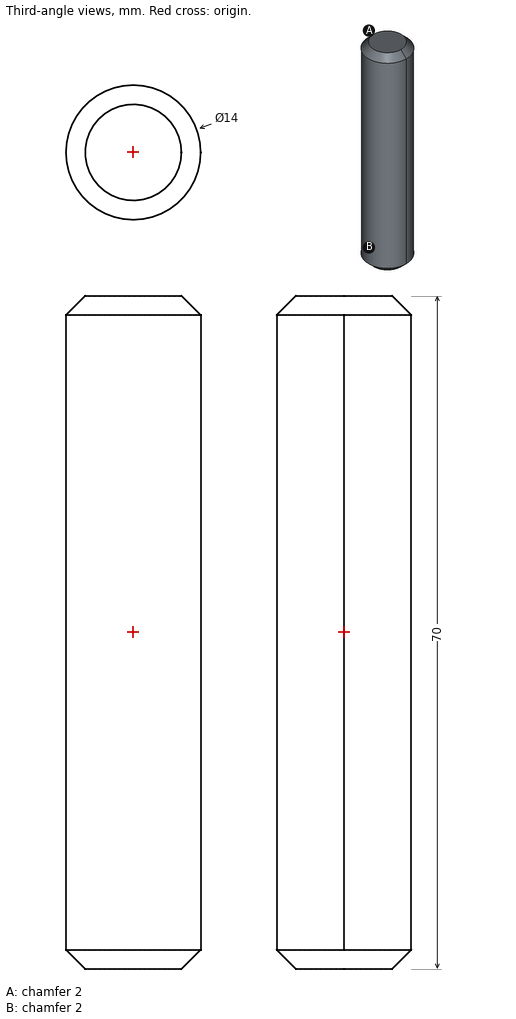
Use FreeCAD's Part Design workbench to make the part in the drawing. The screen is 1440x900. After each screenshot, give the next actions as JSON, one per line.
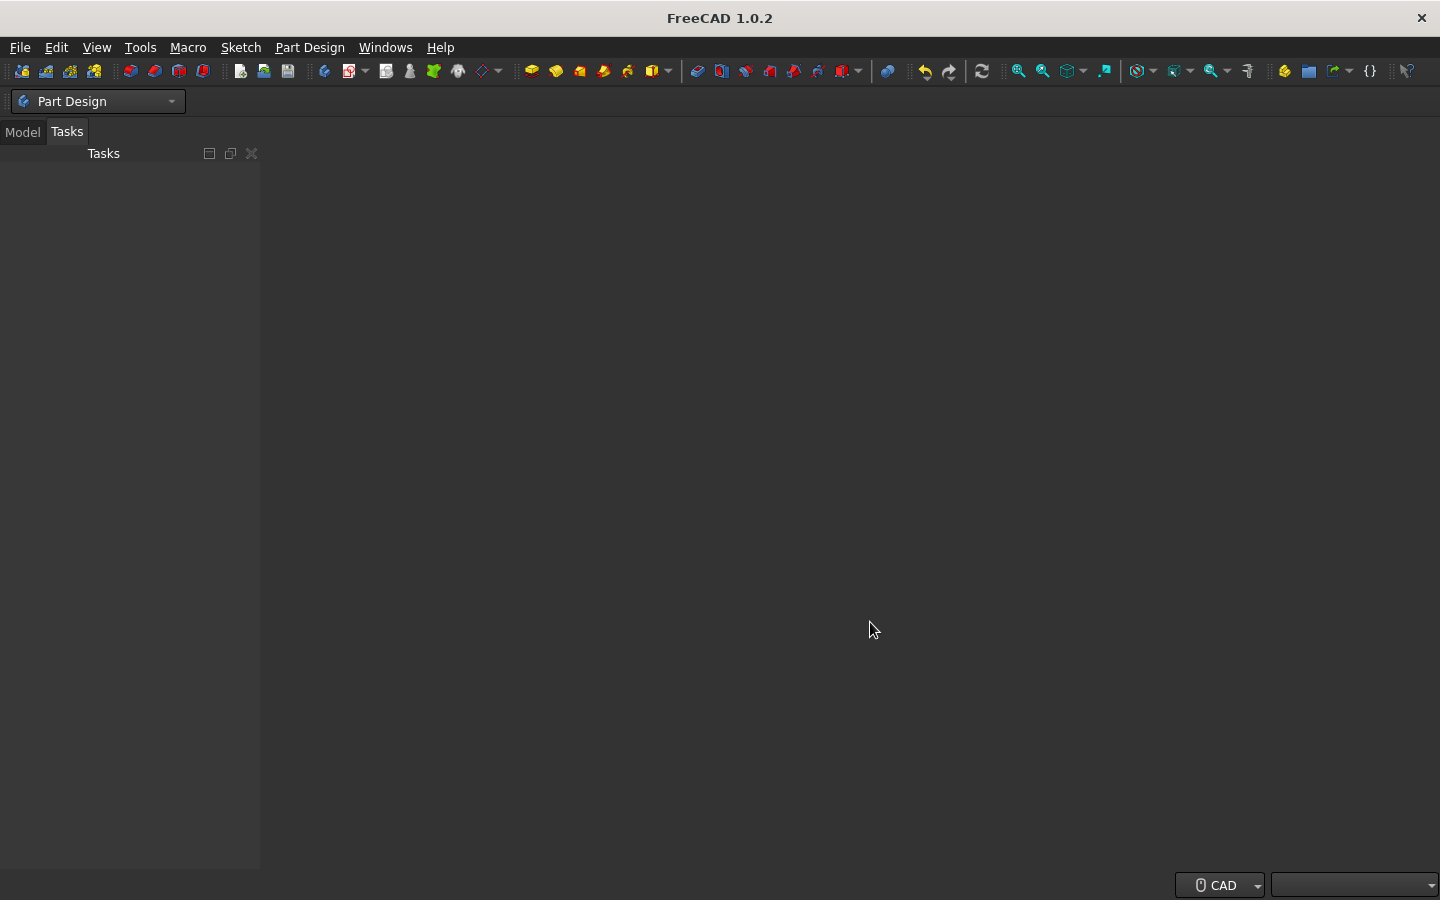
{"action": "key", "text": "ctrl+n"}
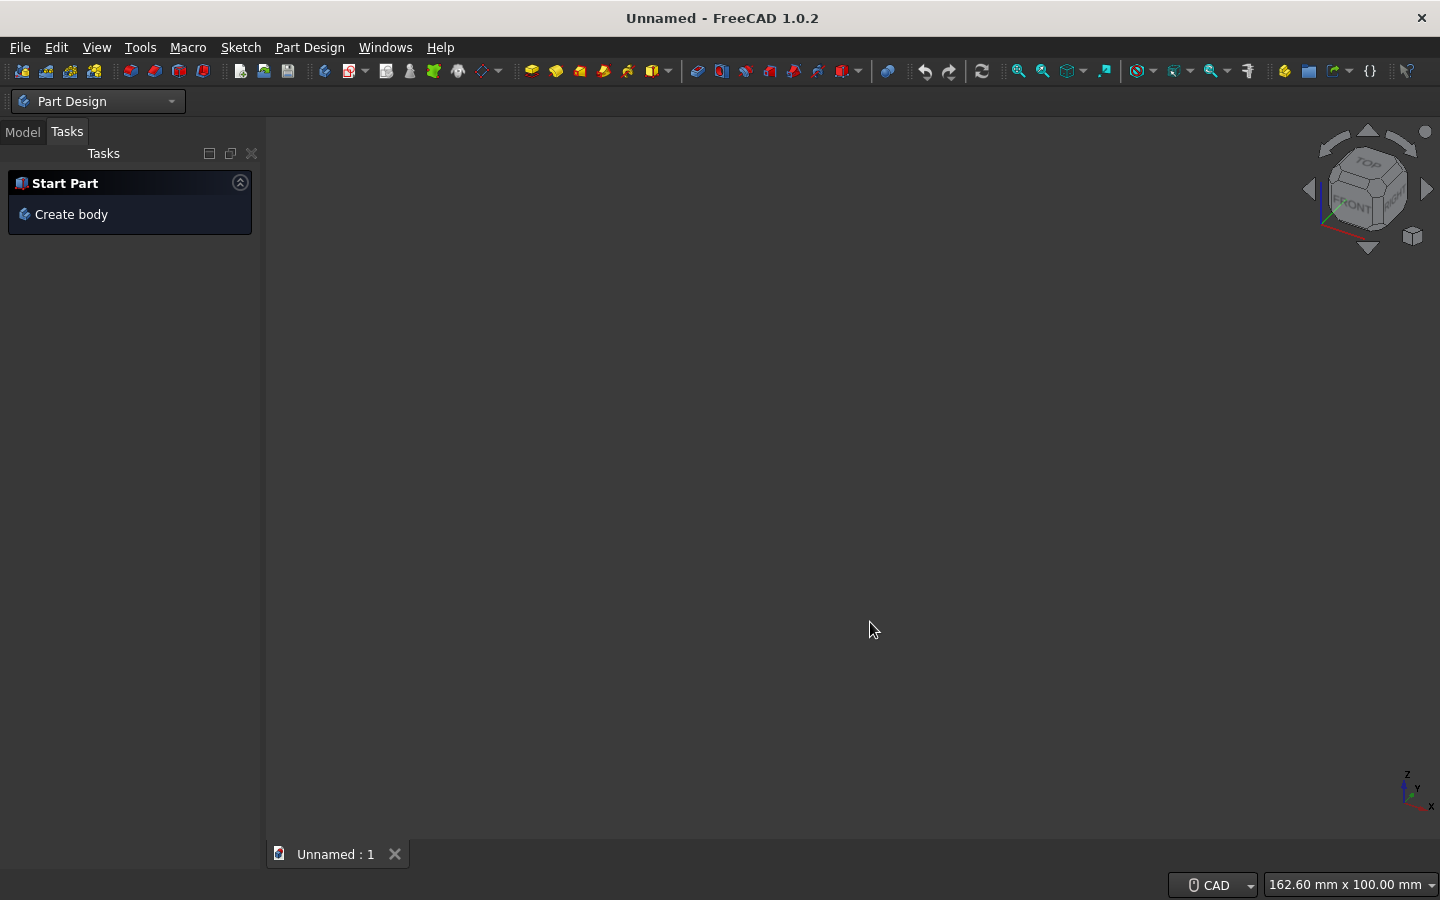
{"action": "left_click", "coordinate": [350, 72]}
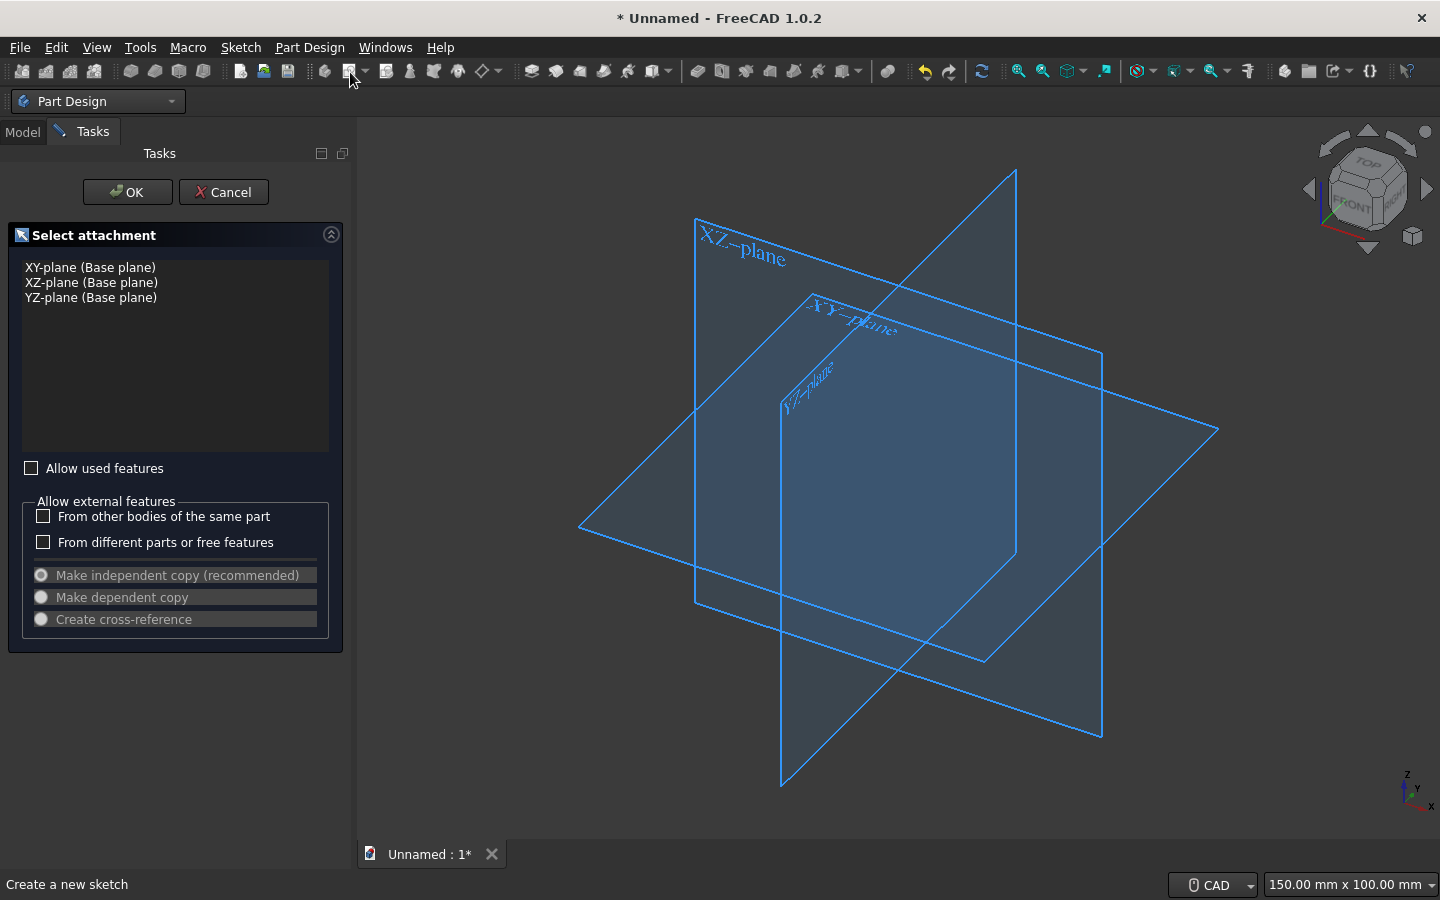
{"action": "left_click", "coordinate": [82, 268]}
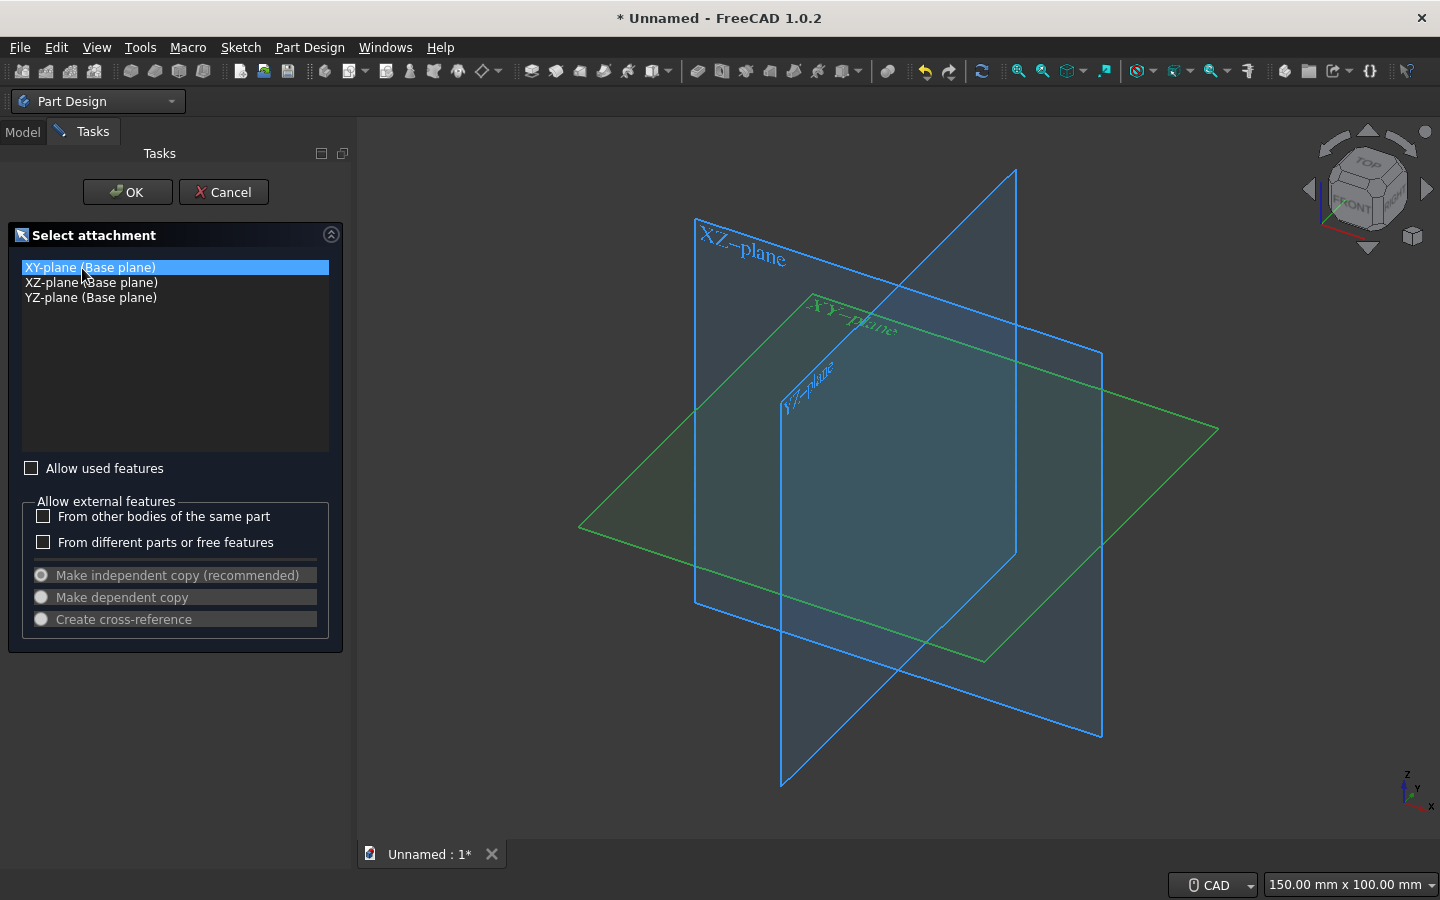
{"action": "left_click", "coordinate": [128, 192]}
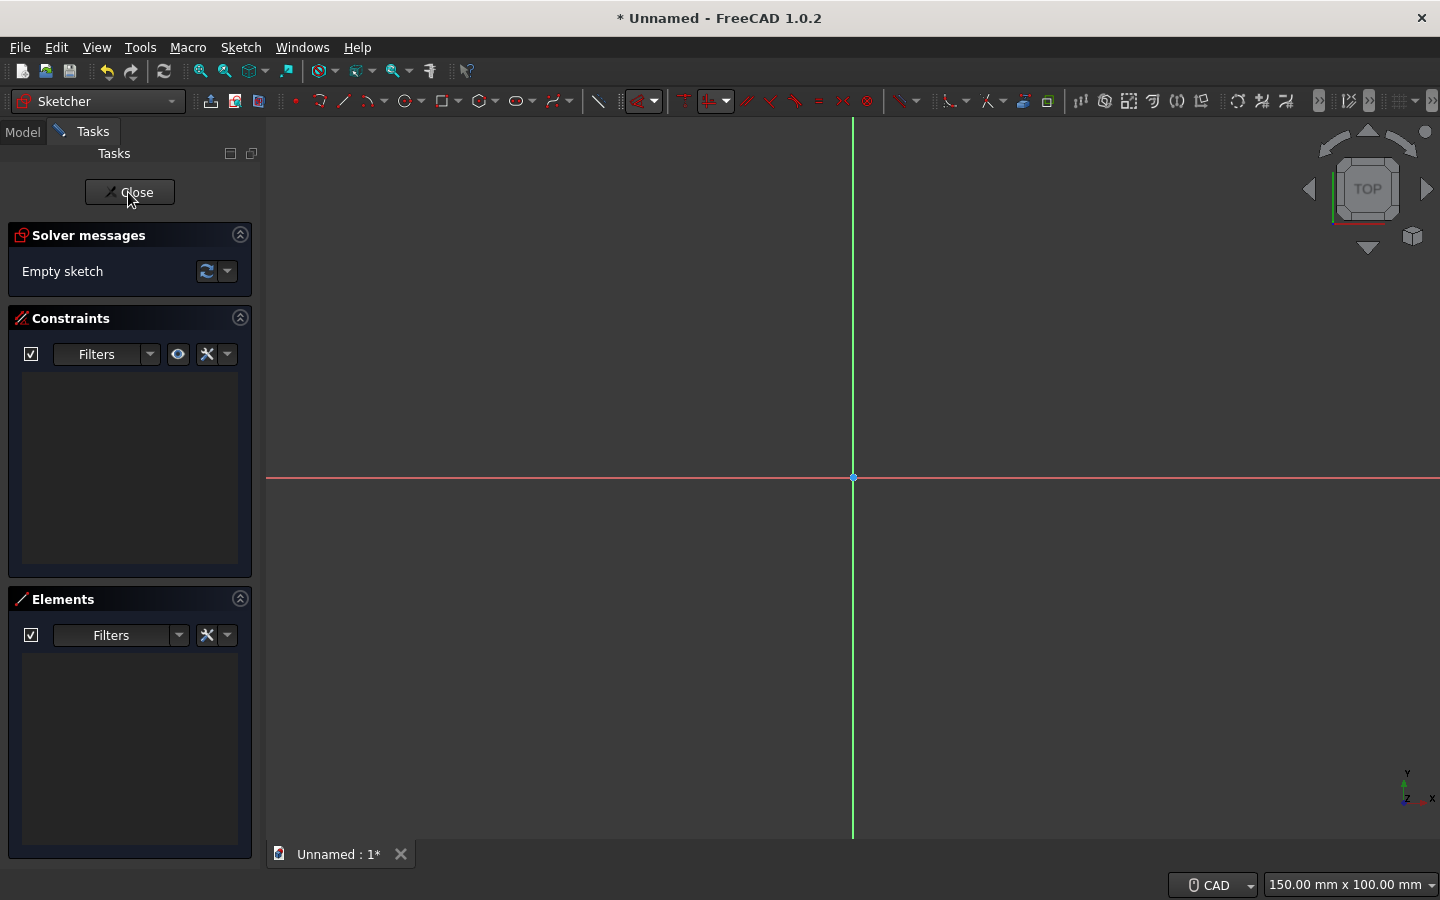
{"action": "scroll", "coordinate": [870, 478], "scroll_direction": "up", "scroll_amount": 8}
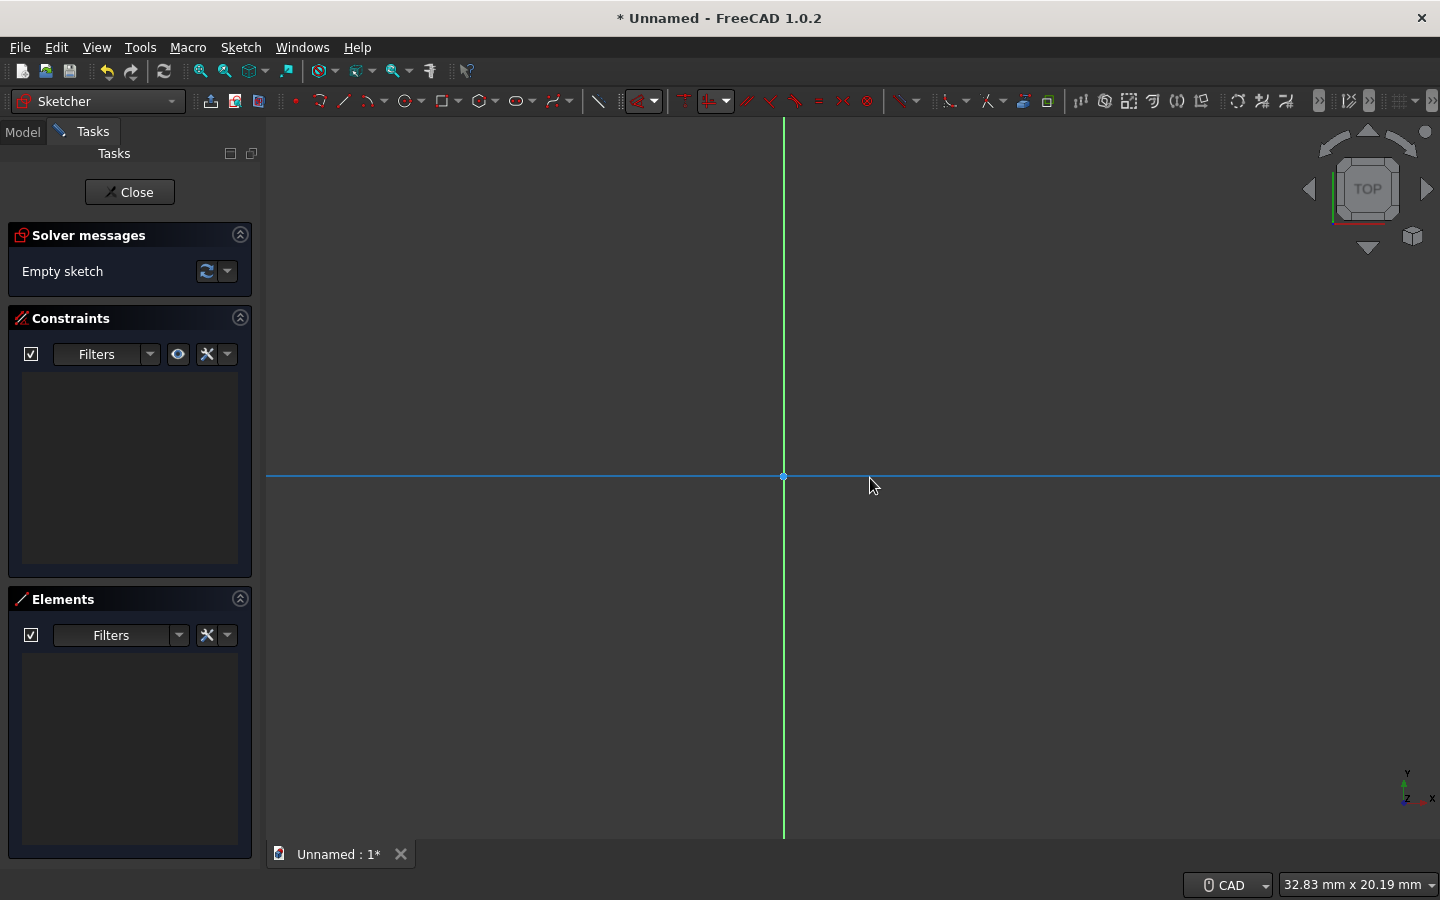
{"action": "key", "text": "g c"}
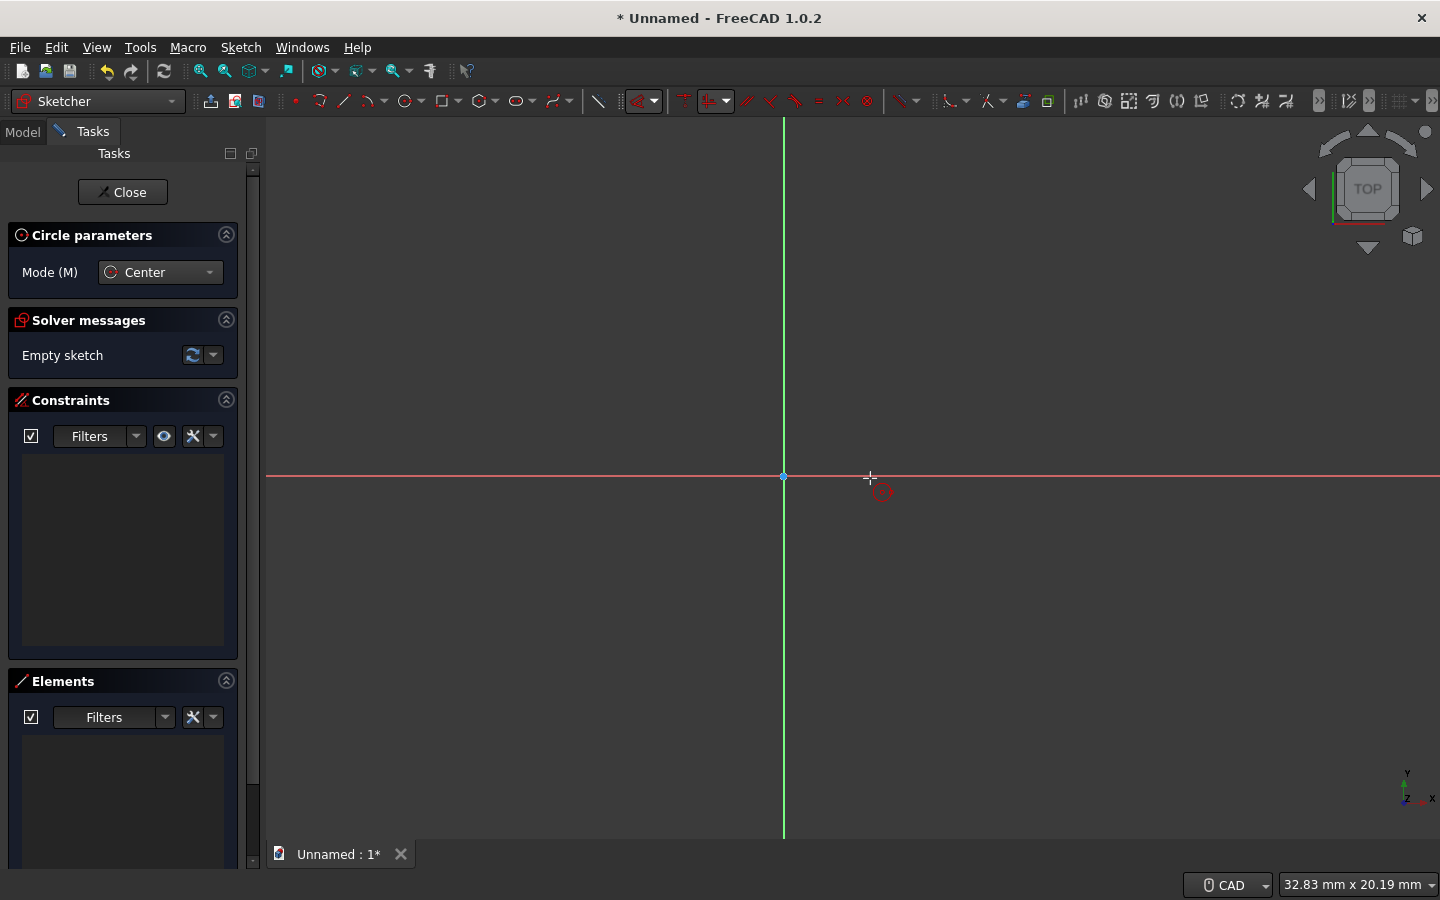
{"action": "left_click", "coordinate": [784, 476]}
{"action": "left_click", "coordinate": [961, 299]}
{"action": "key", "text": "Escape"}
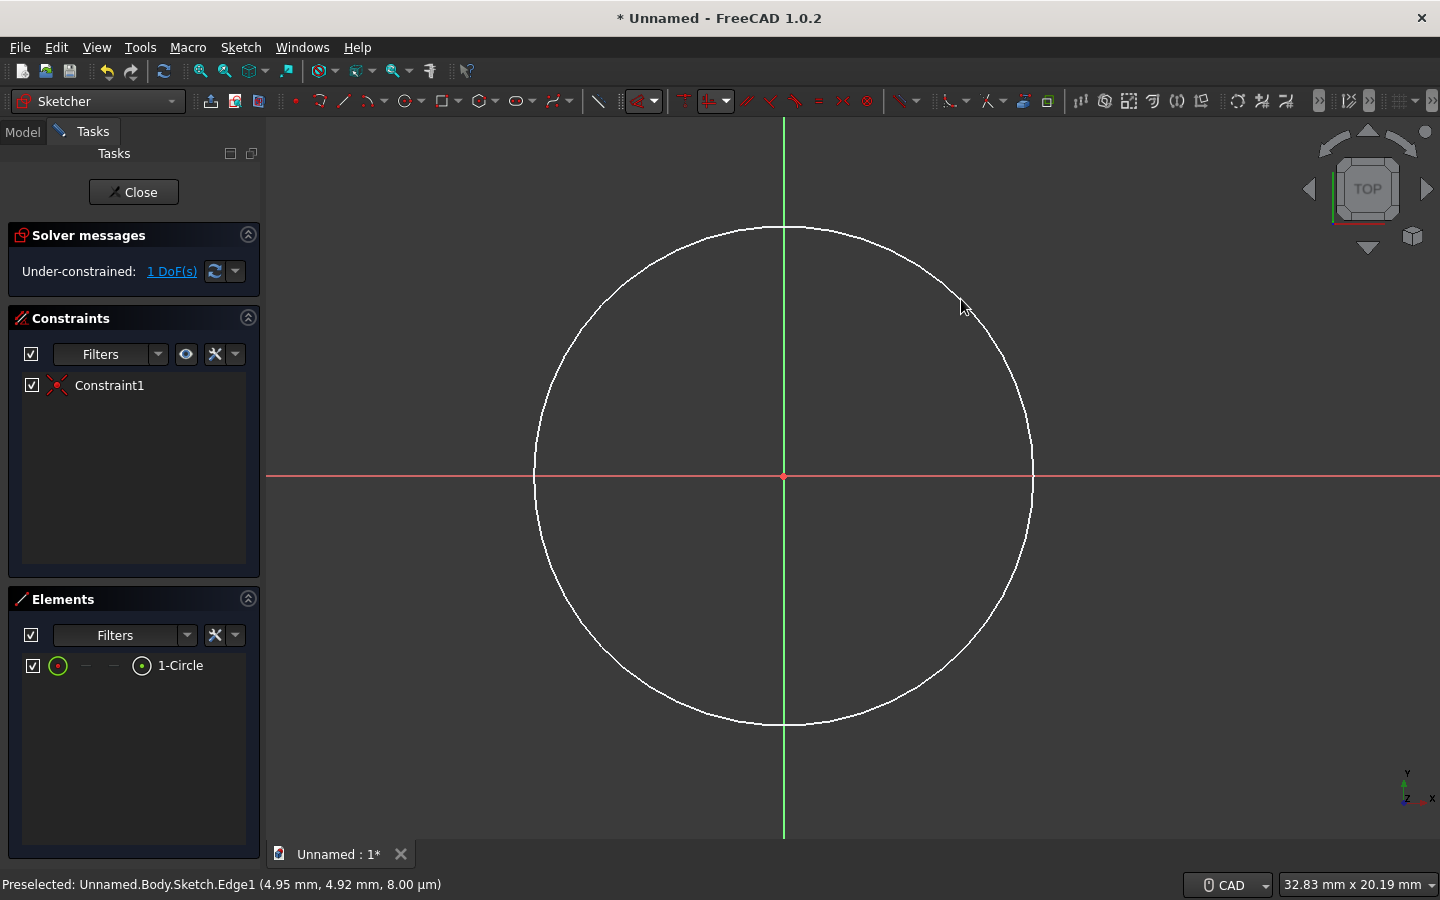
{"action": "left_click", "coordinate": [960, 299]}